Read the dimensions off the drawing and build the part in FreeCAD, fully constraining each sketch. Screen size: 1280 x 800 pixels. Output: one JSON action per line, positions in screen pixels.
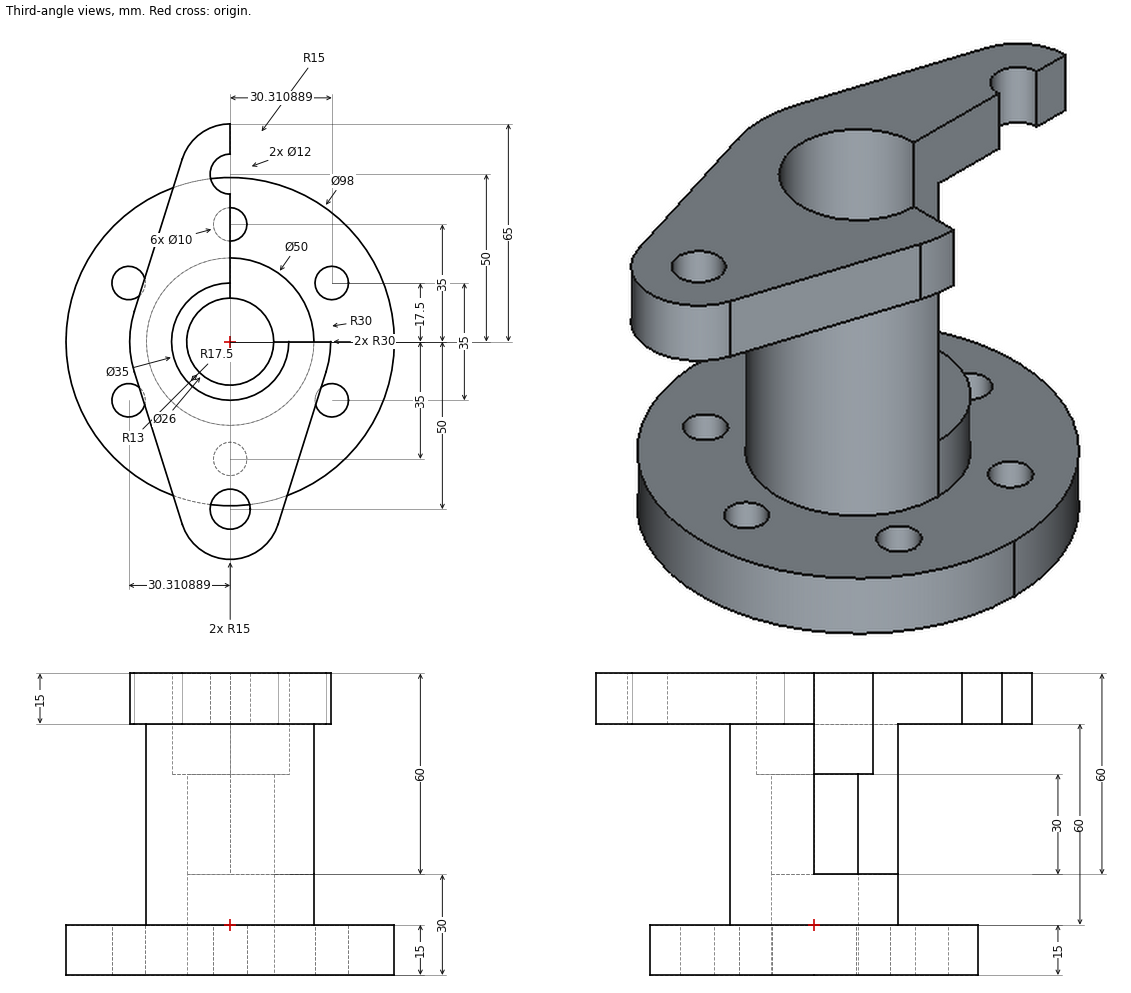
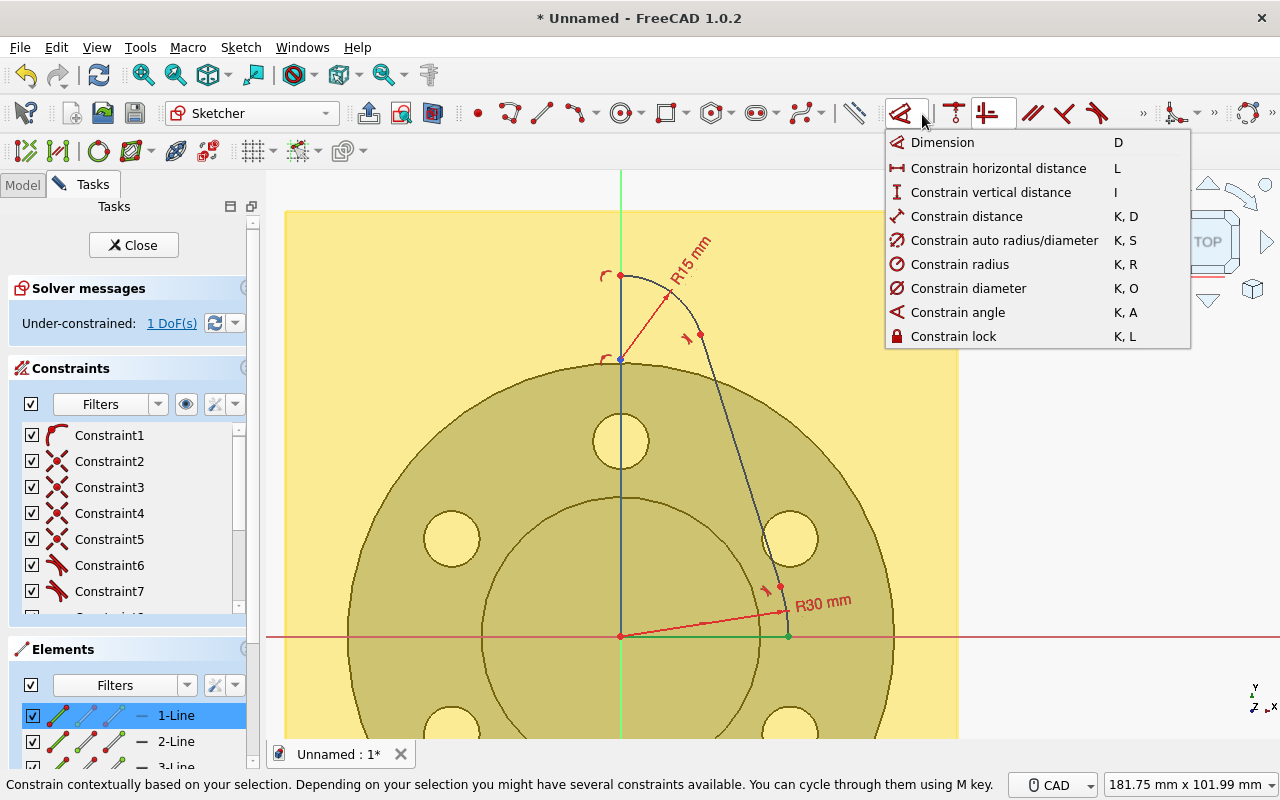
{"action": "left_click", "coordinate": [1038, 192]}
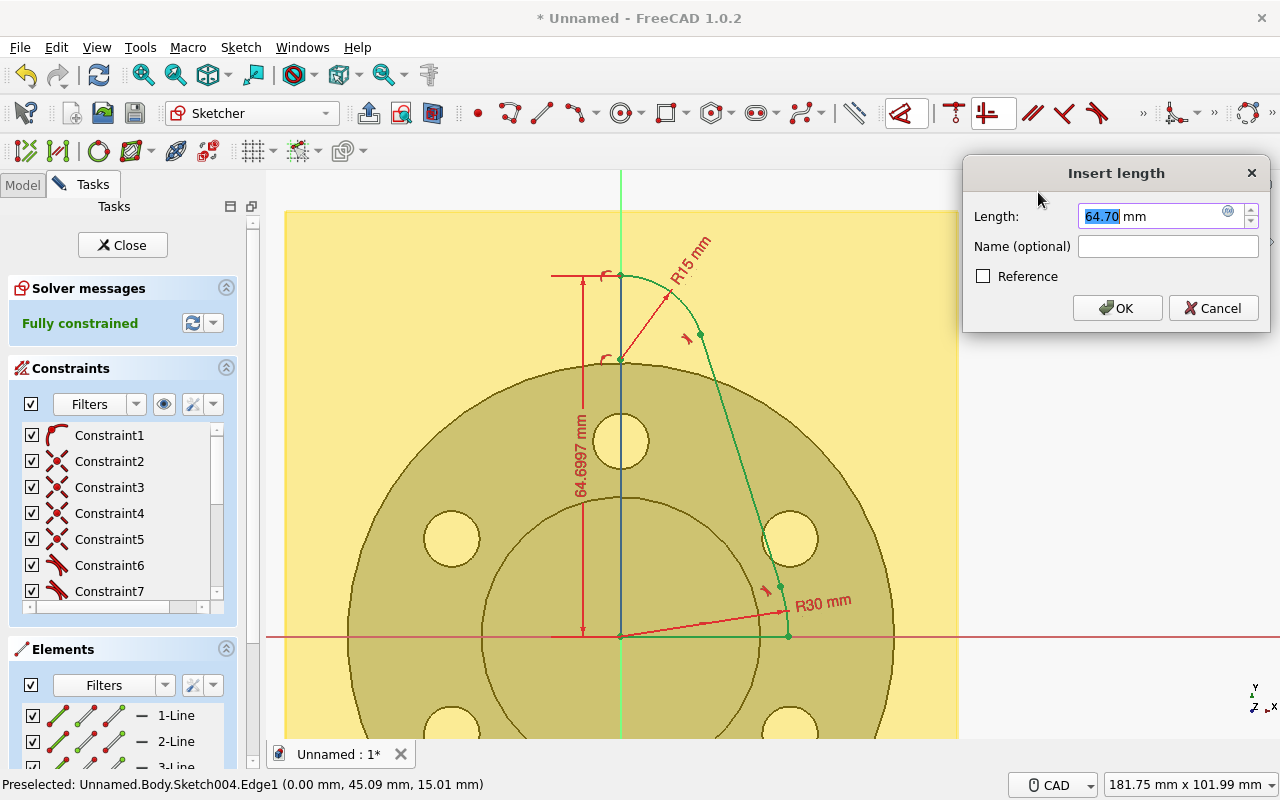
{"action": "type", "text": "65"}
{"action": "key", "text": "Return"}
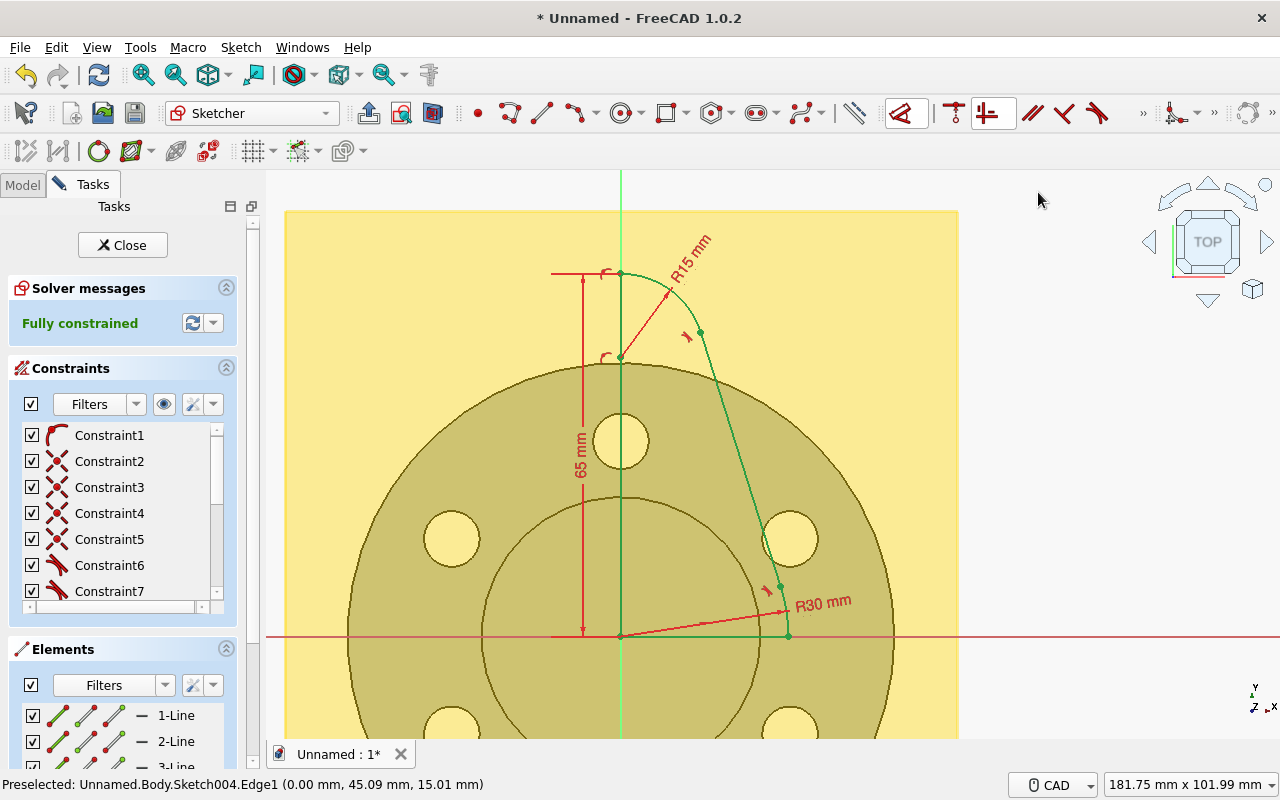
{"action": "left_click", "coordinate": [123, 245]}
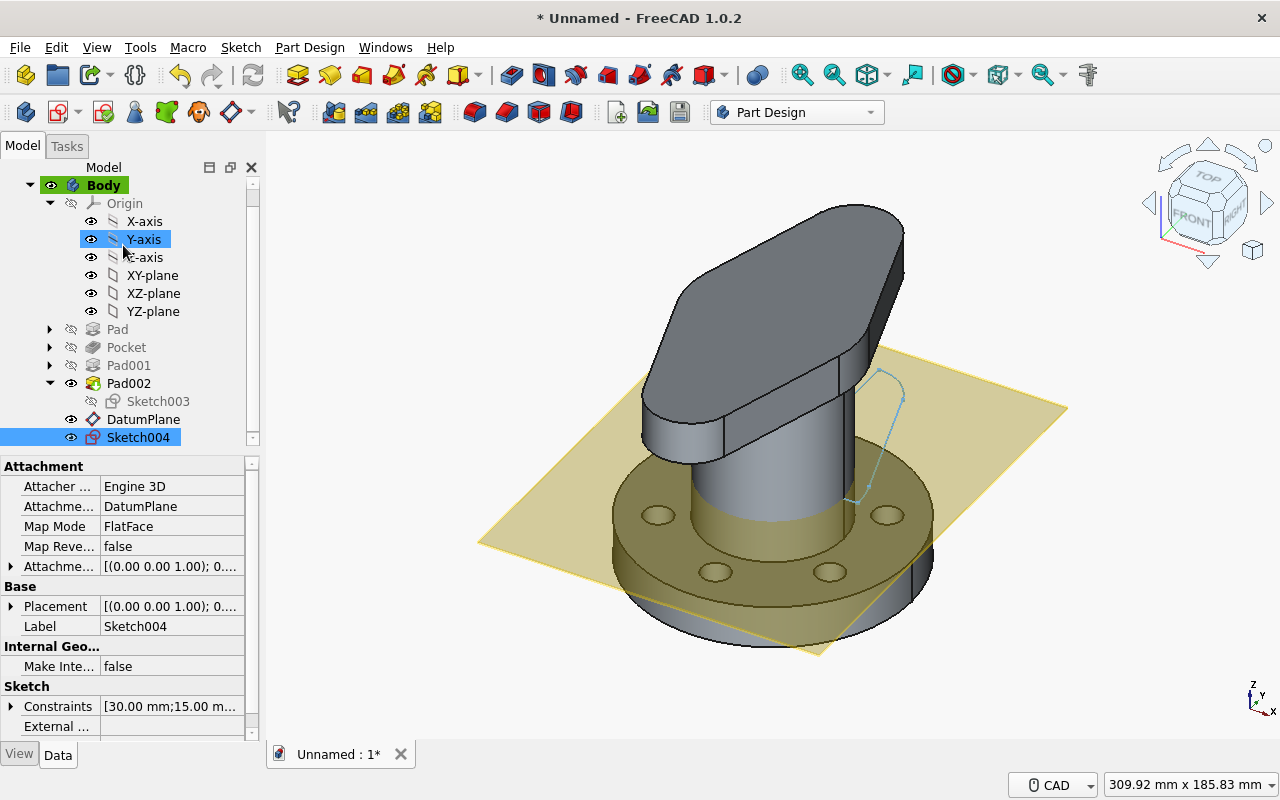
{"action": "left_click", "coordinate": [512, 76]}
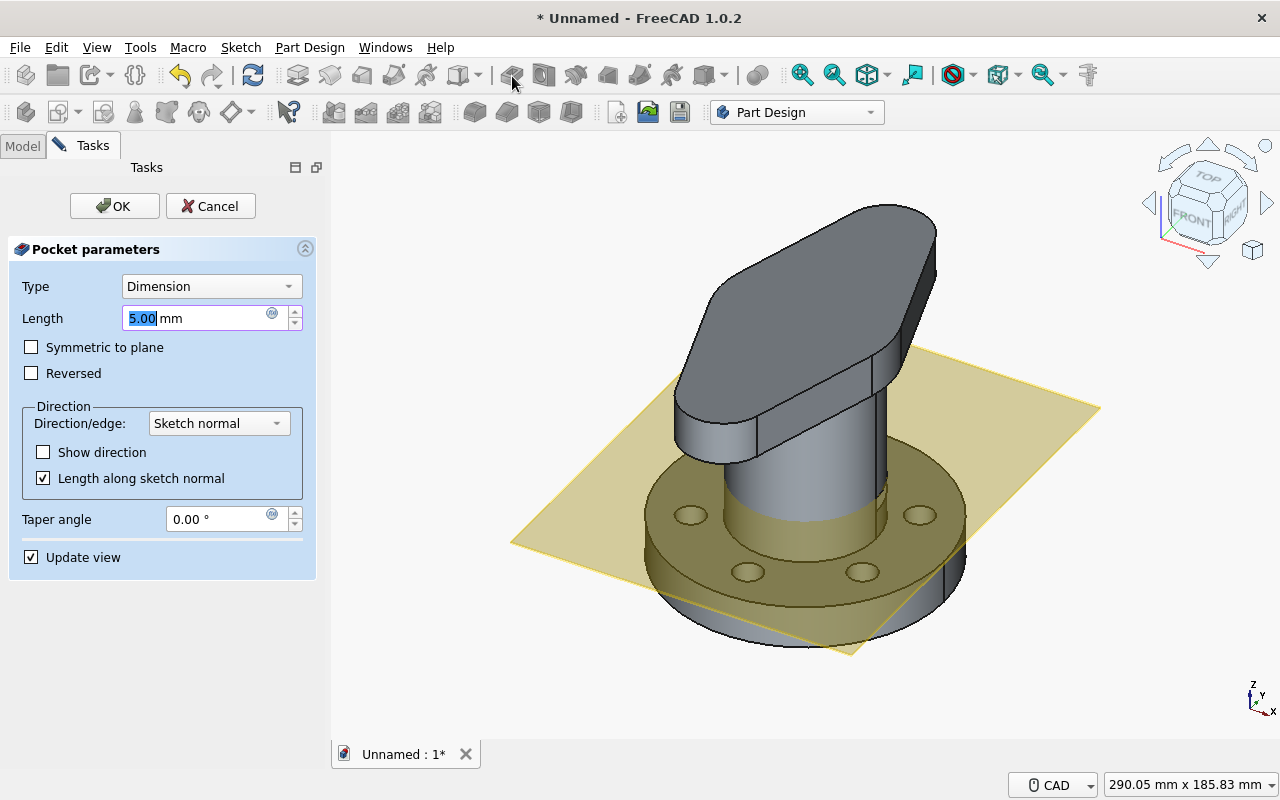
{"action": "type", "text": "60"}
{"action": "key", "text": "Tab"}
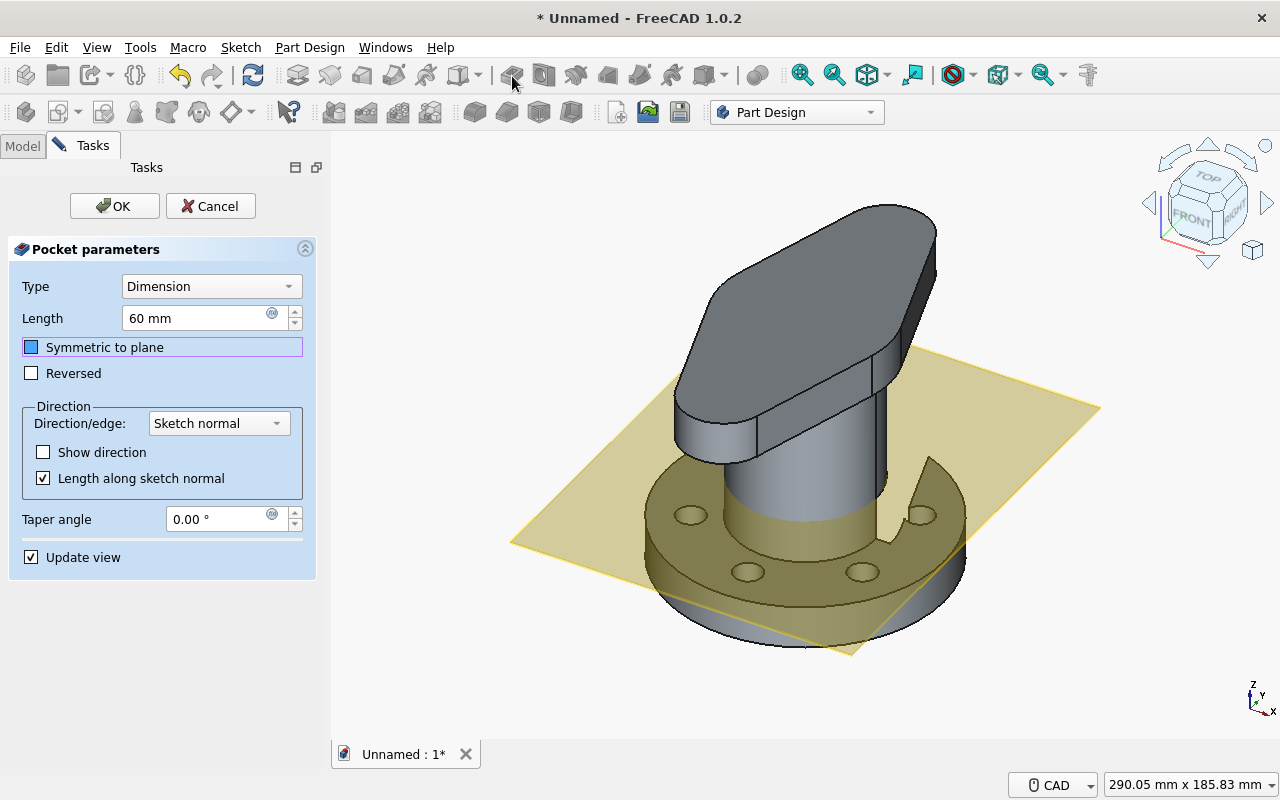
{"action": "left_click", "coordinate": [30, 373]}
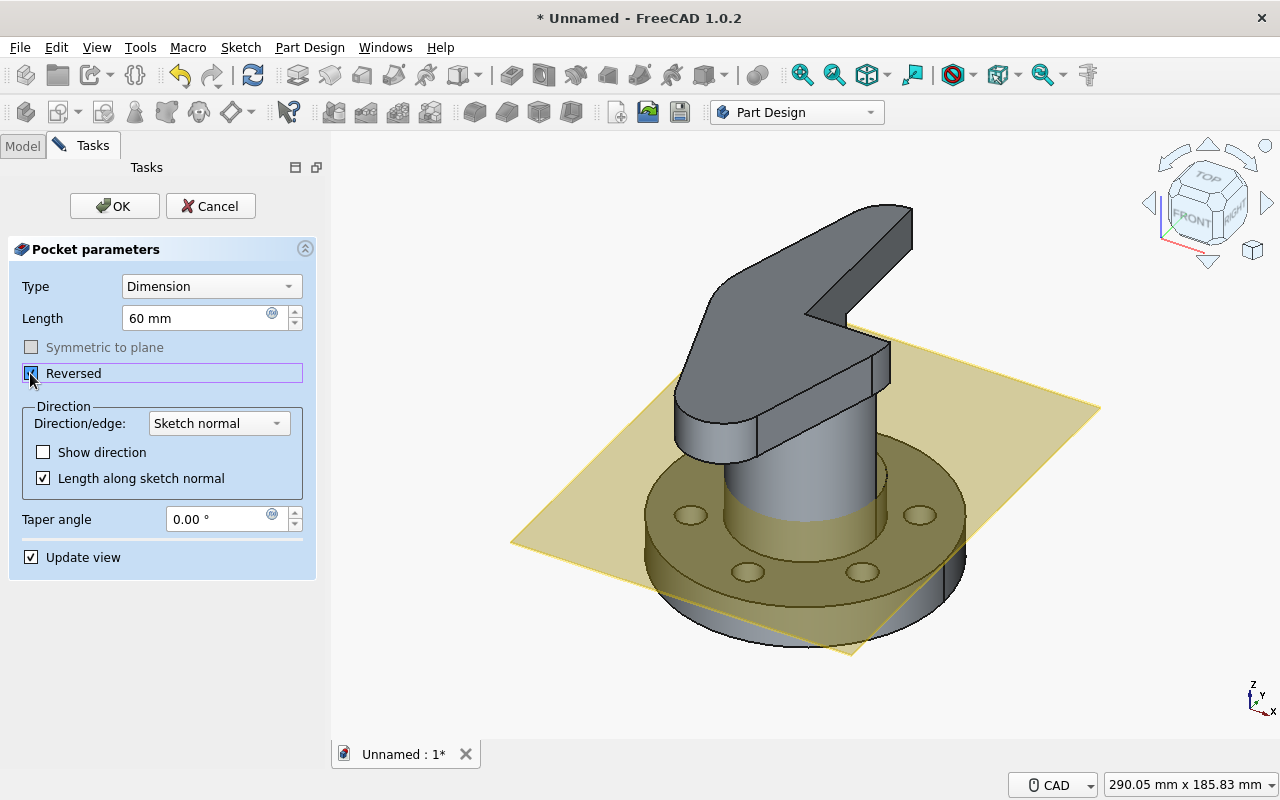
{"action": "left_click", "coordinate": [115, 206]}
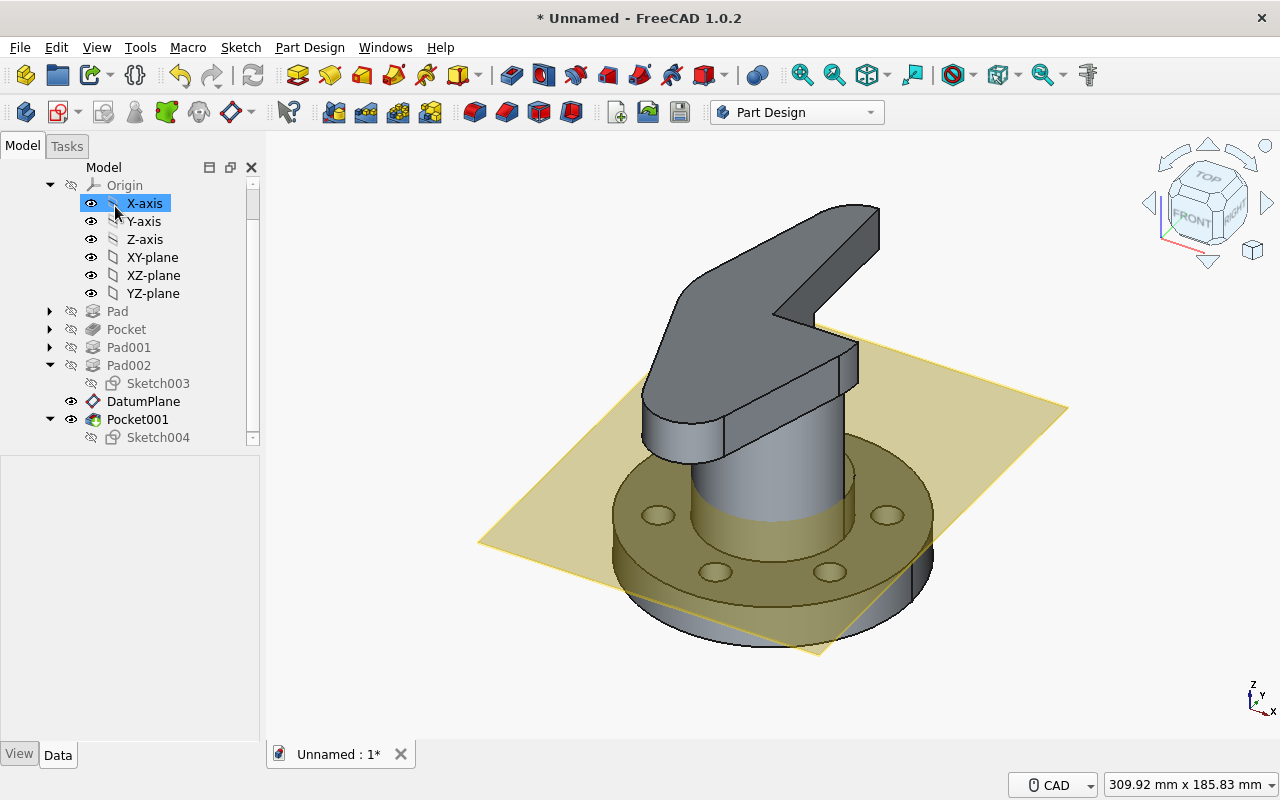
{"action": "left_click", "coordinate": [116, 401]}
{"action": "key", "text": "space"}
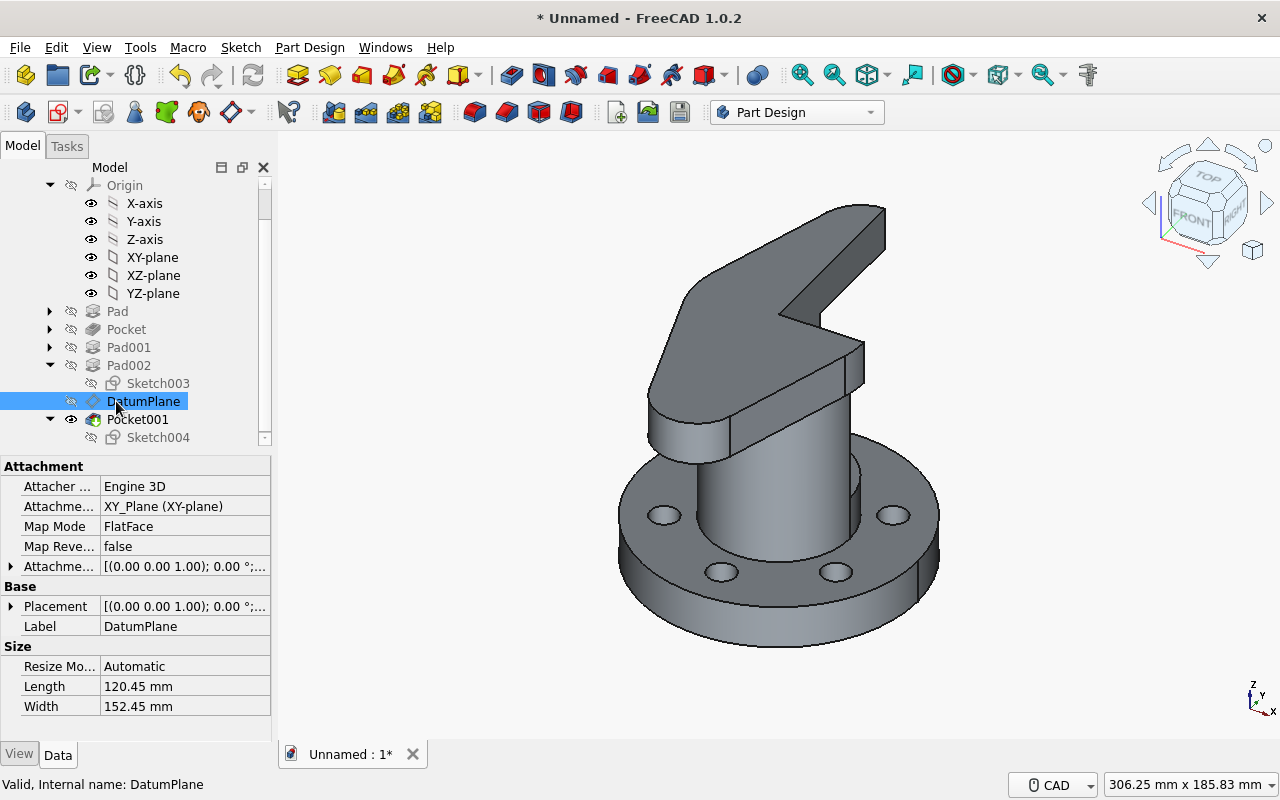
{"action": "left_click", "coordinate": [718, 374]}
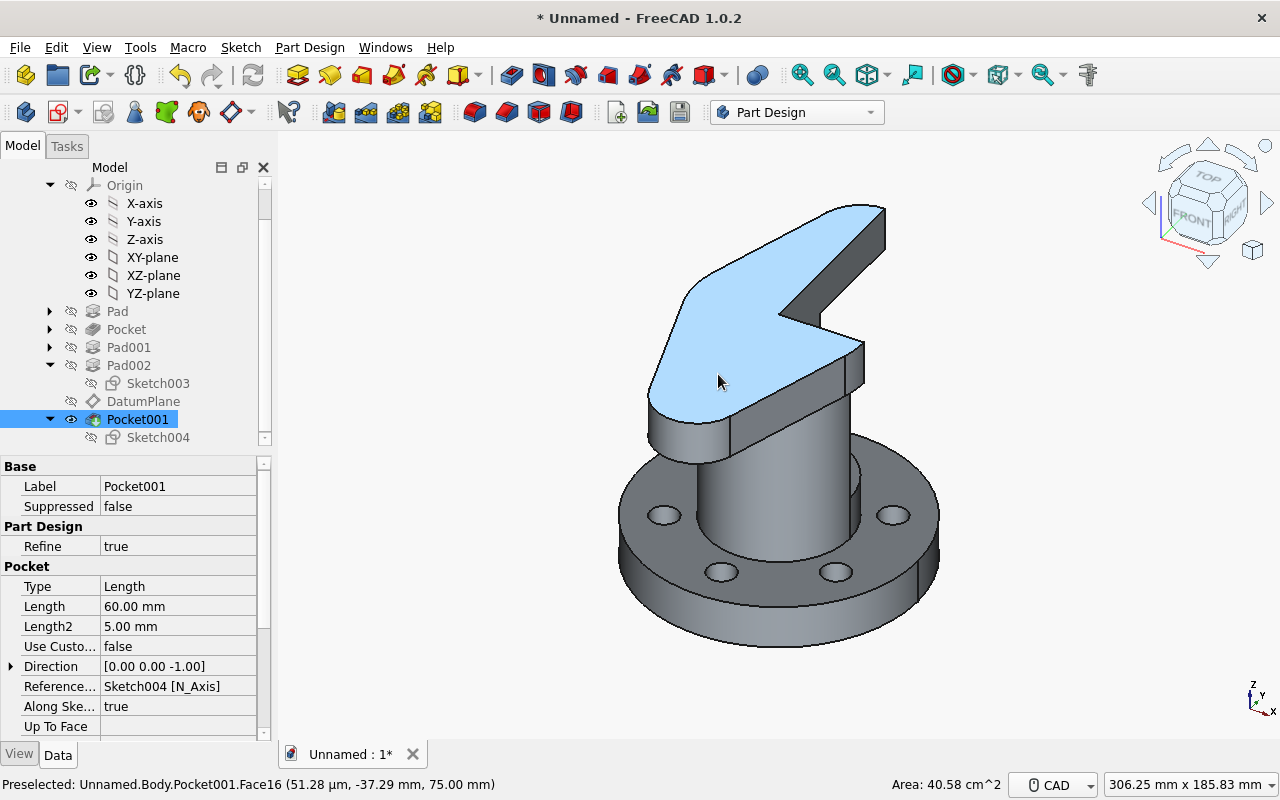
{"action": "left_click", "coordinate": [58, 112]}